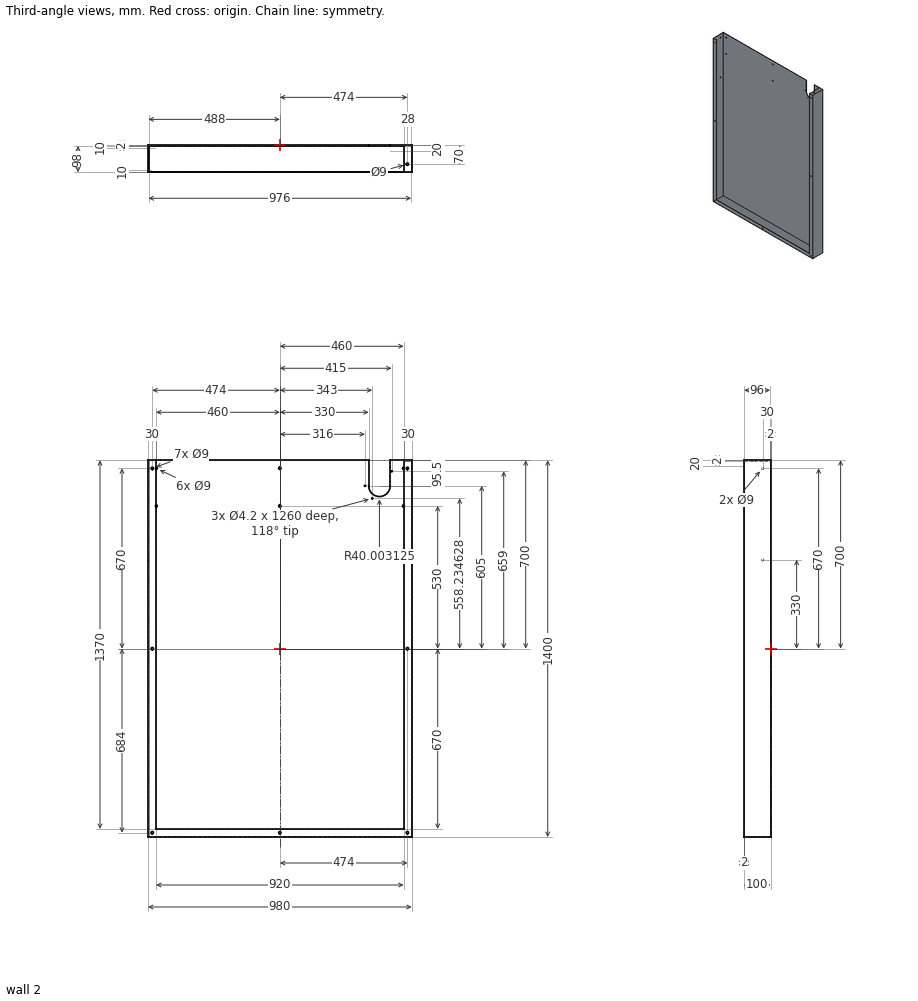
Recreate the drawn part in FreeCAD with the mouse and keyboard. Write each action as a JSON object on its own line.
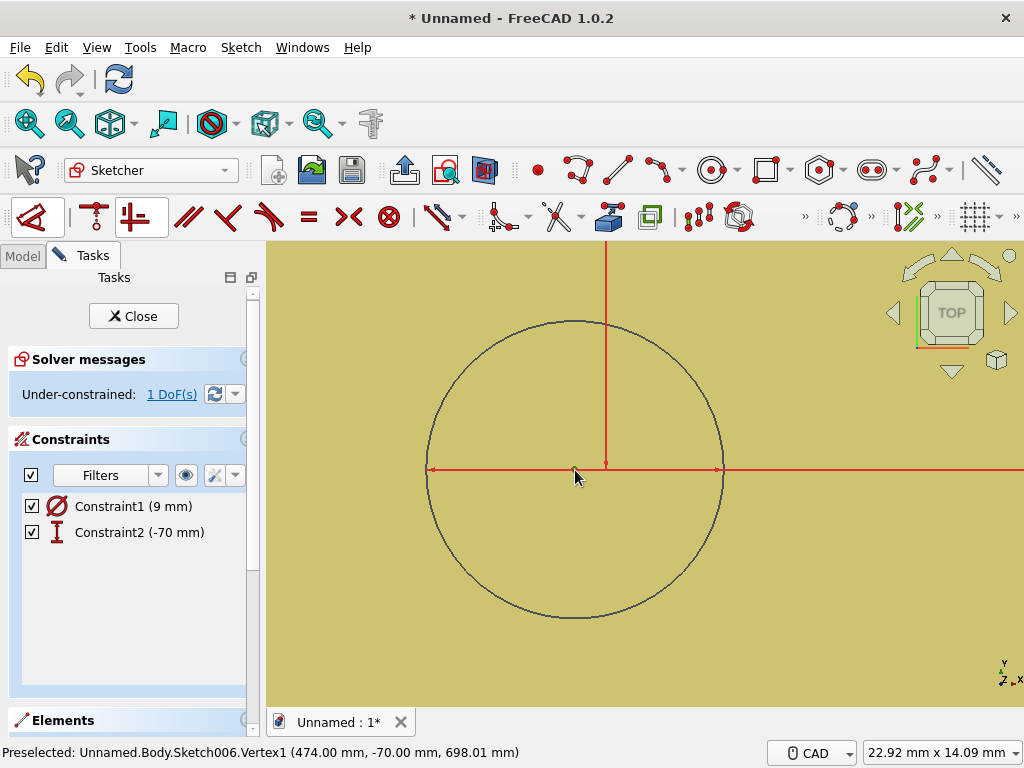
{"action": "left_click", "coordinate": [58, 218]}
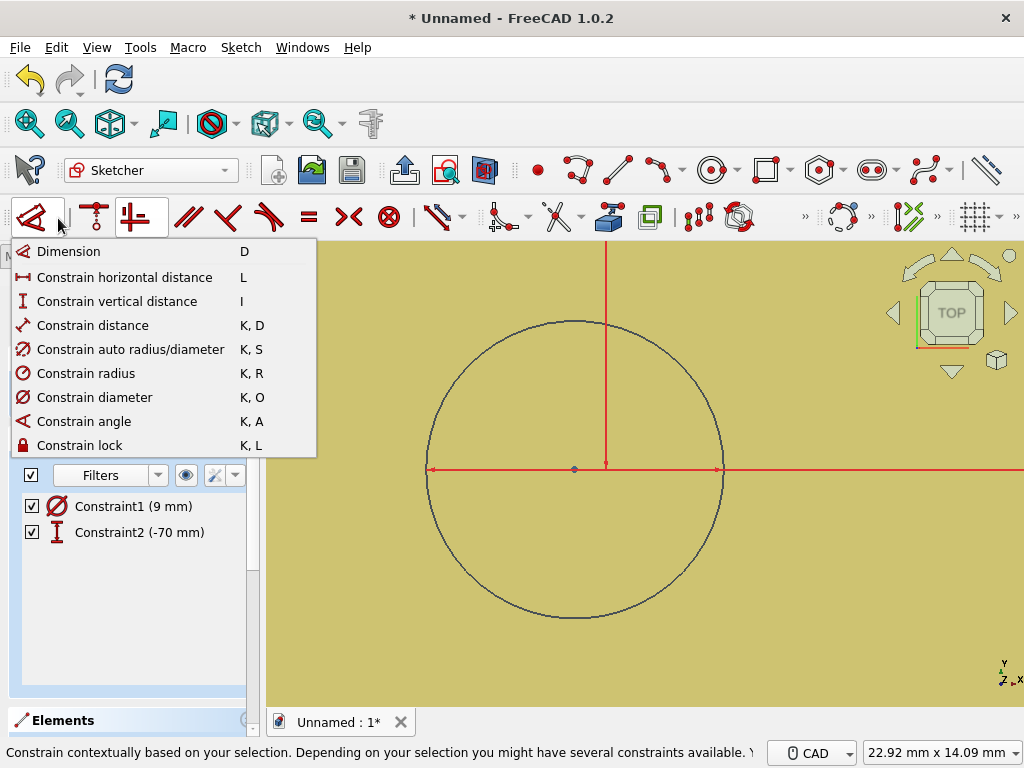
{"action": "left_click", "coordinate": [164, 277]}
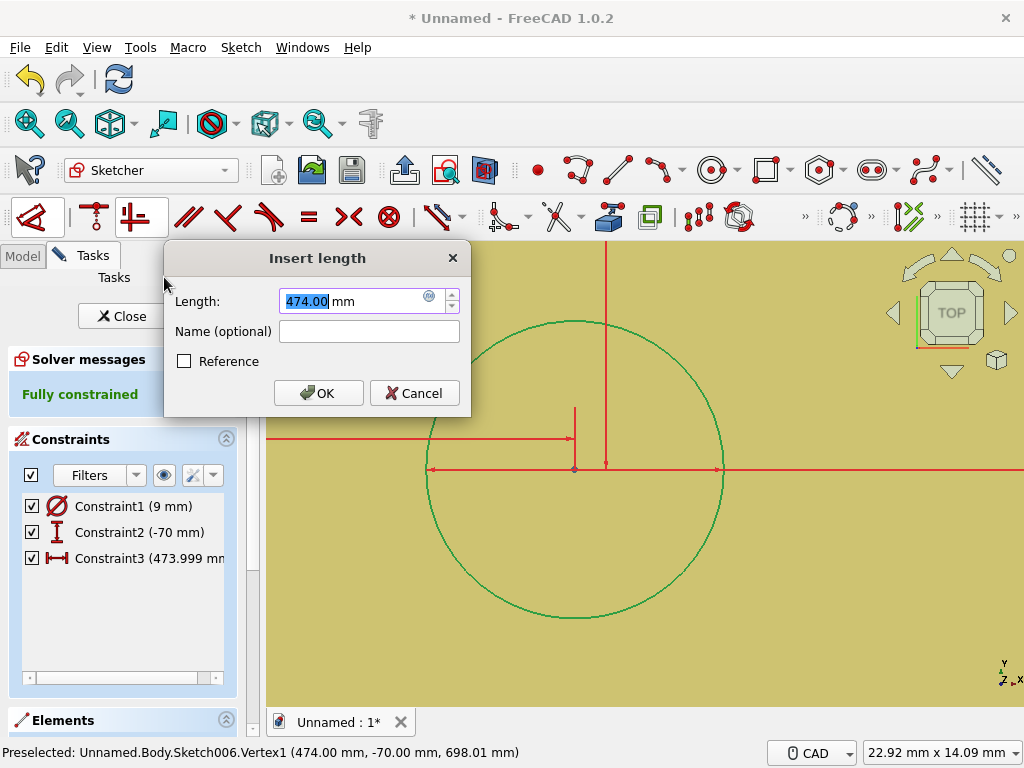
{"action": "type", "text": "474"}
{"action": "key", "text": "Return"}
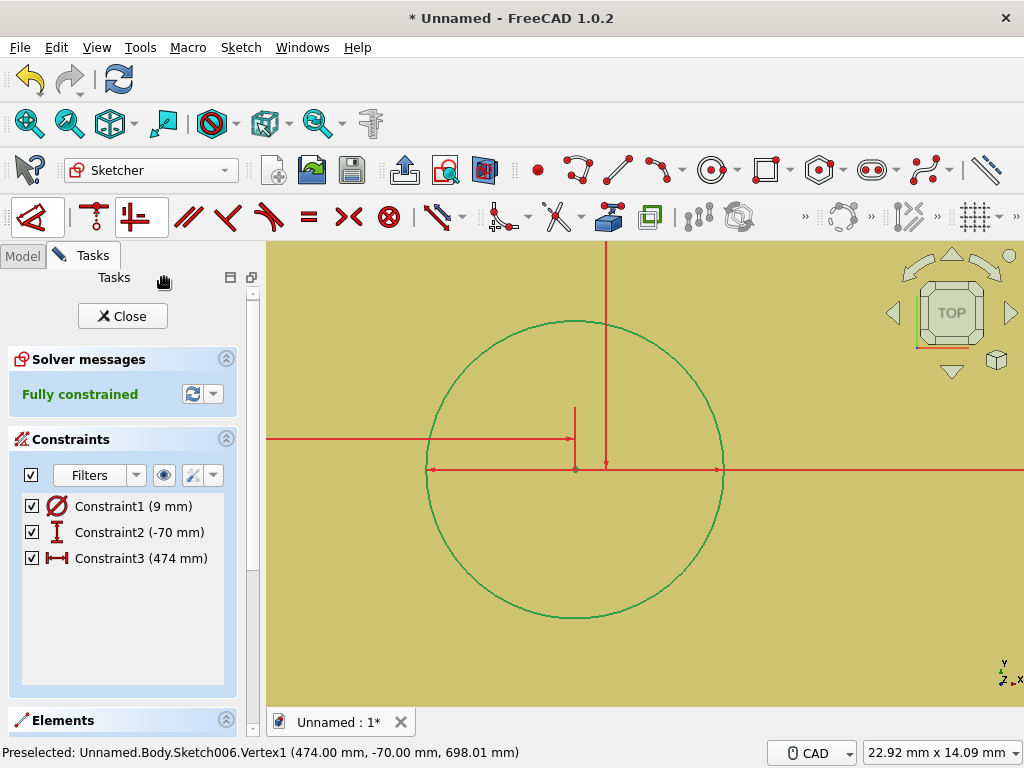
{"action": "left_click", "coordinate": [123, 316]}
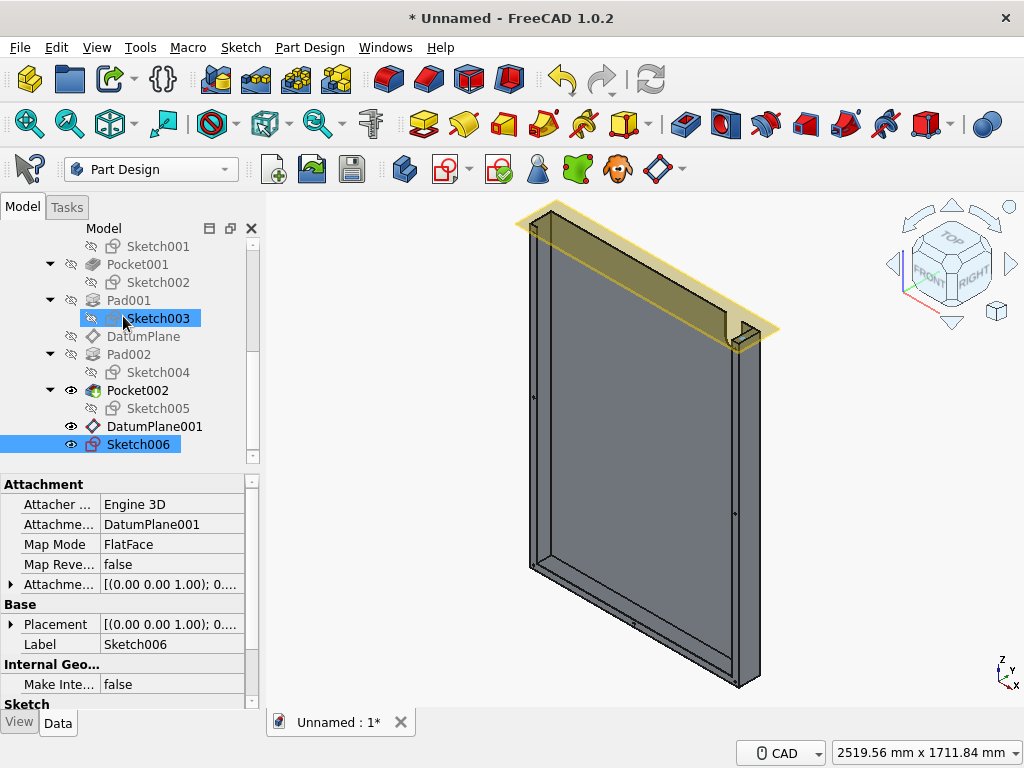
{"action": "left_click", "coordinate": [686, 124]}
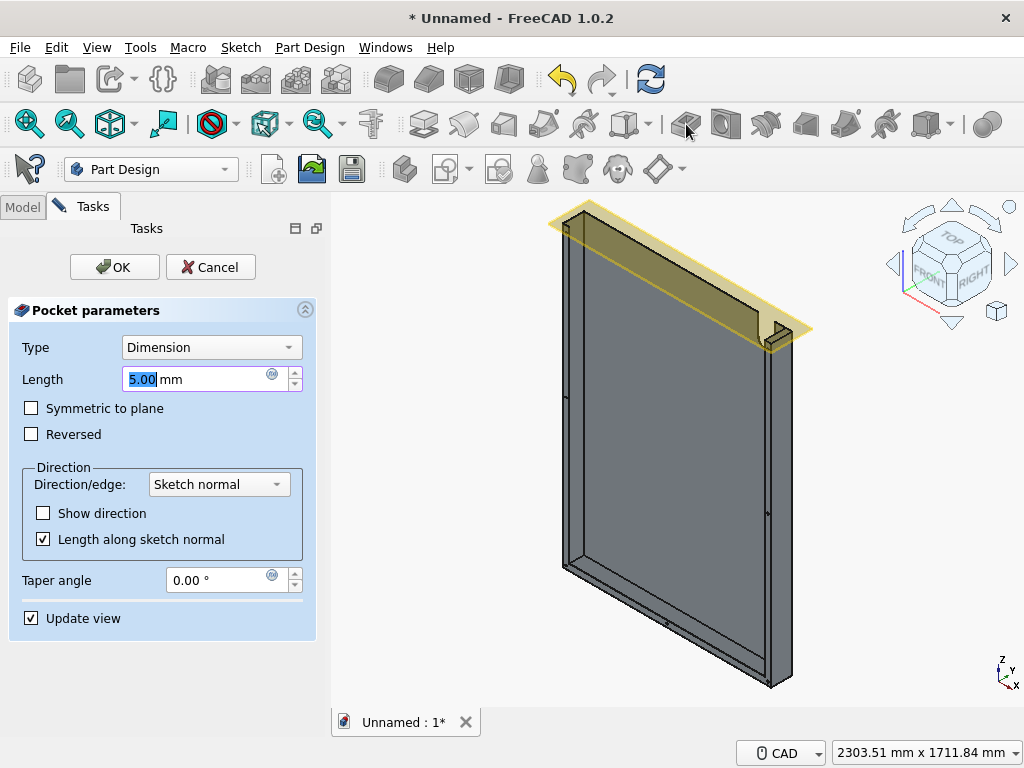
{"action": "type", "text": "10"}
{"action": "key", "text": "Tab"}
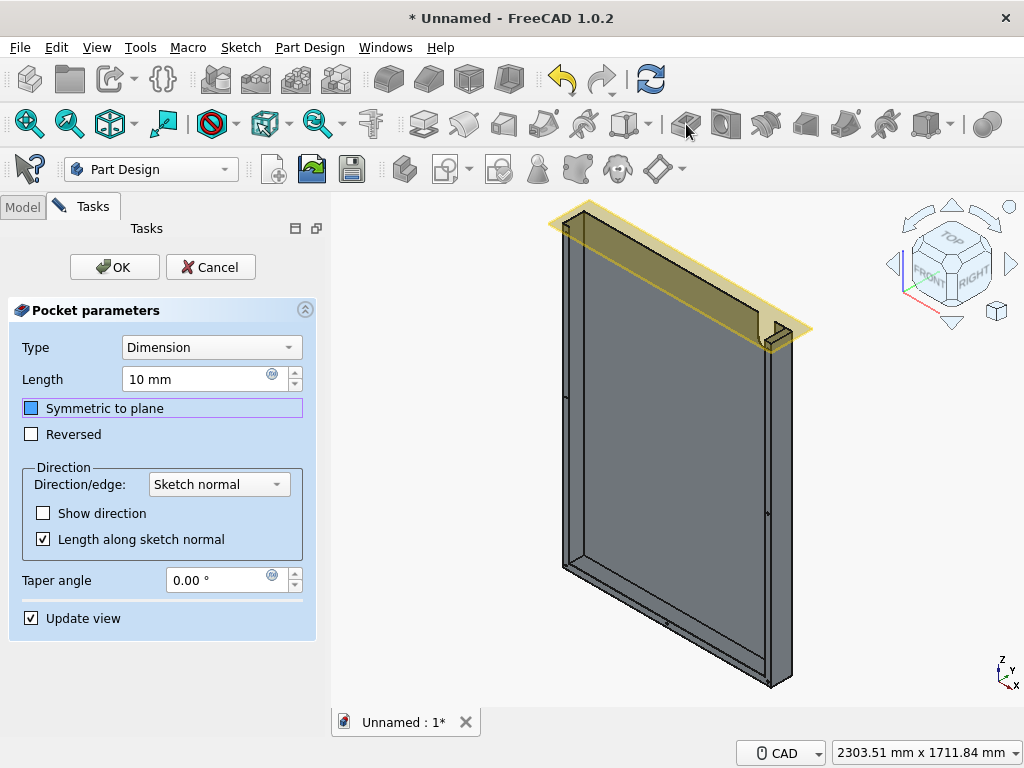
{"action": "left_click", "coordinate": [30, 434]}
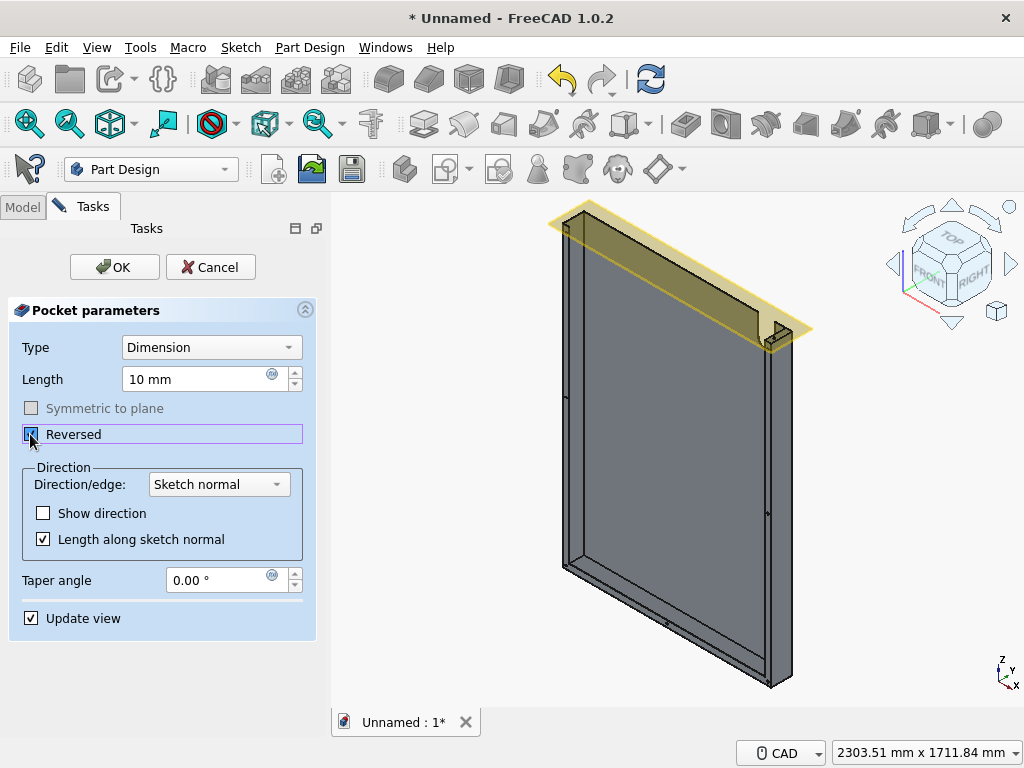
{"action": "left_click", "coordinate": [115, 267]}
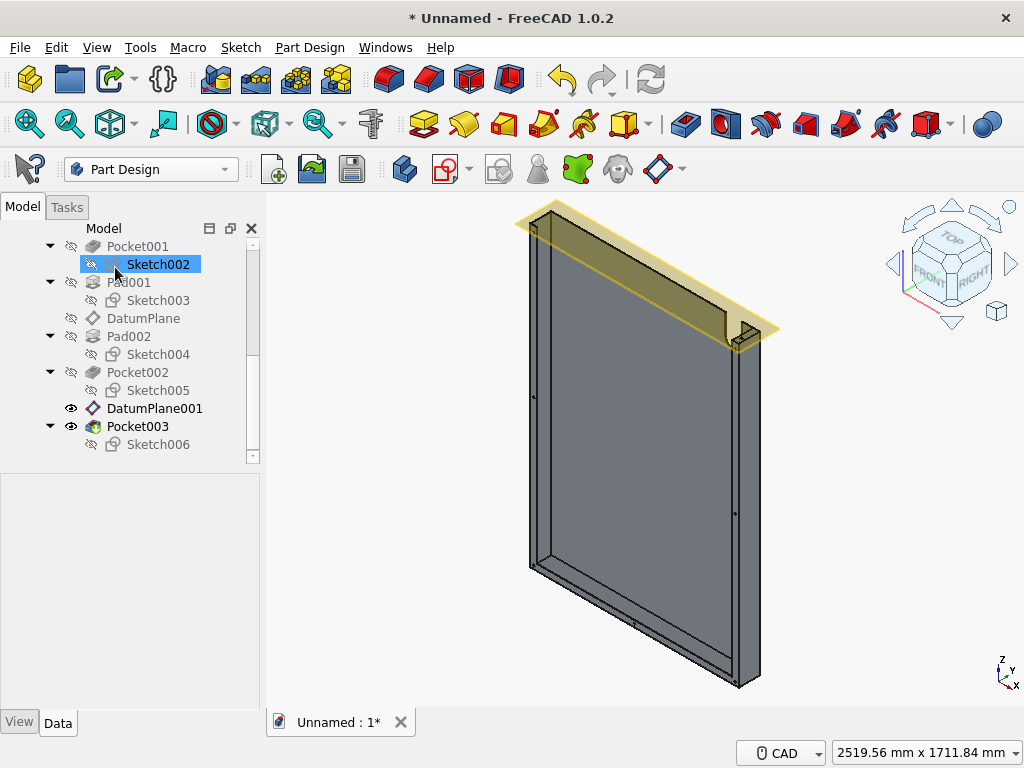
{"action": "left_click", "coordinate": [116, 408]}
{"action": "key", "text": "space"}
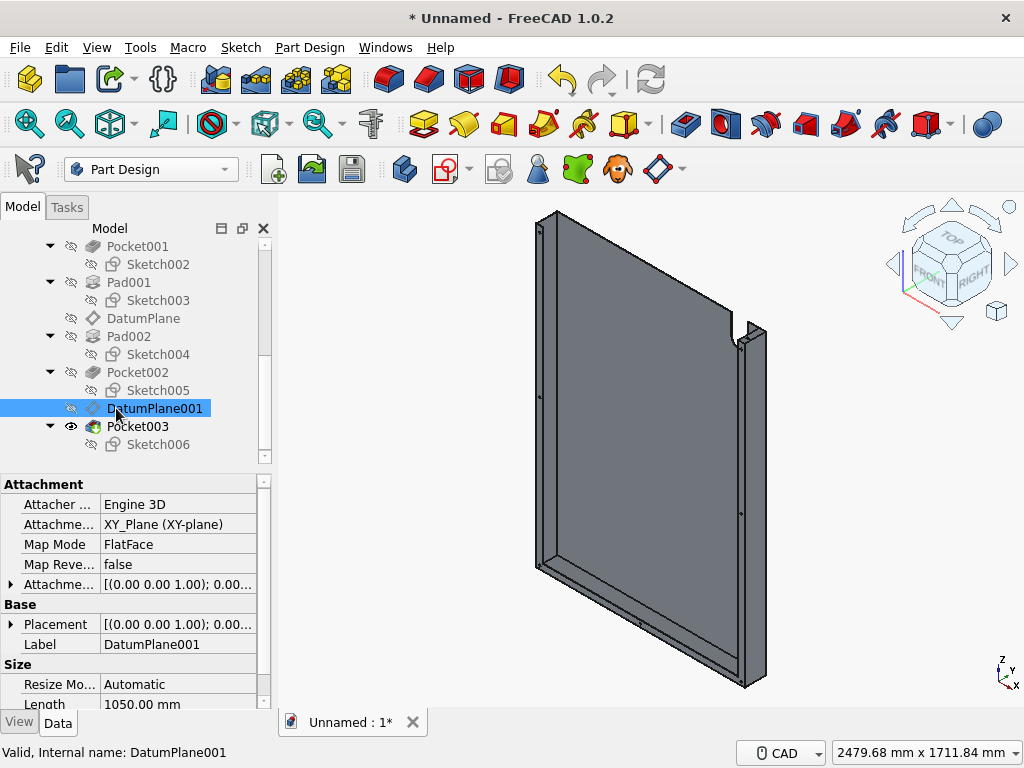
{"action": "scroll", "coordinate": [140, 350], "scroll_direction": "down", "scroll_amount": 3}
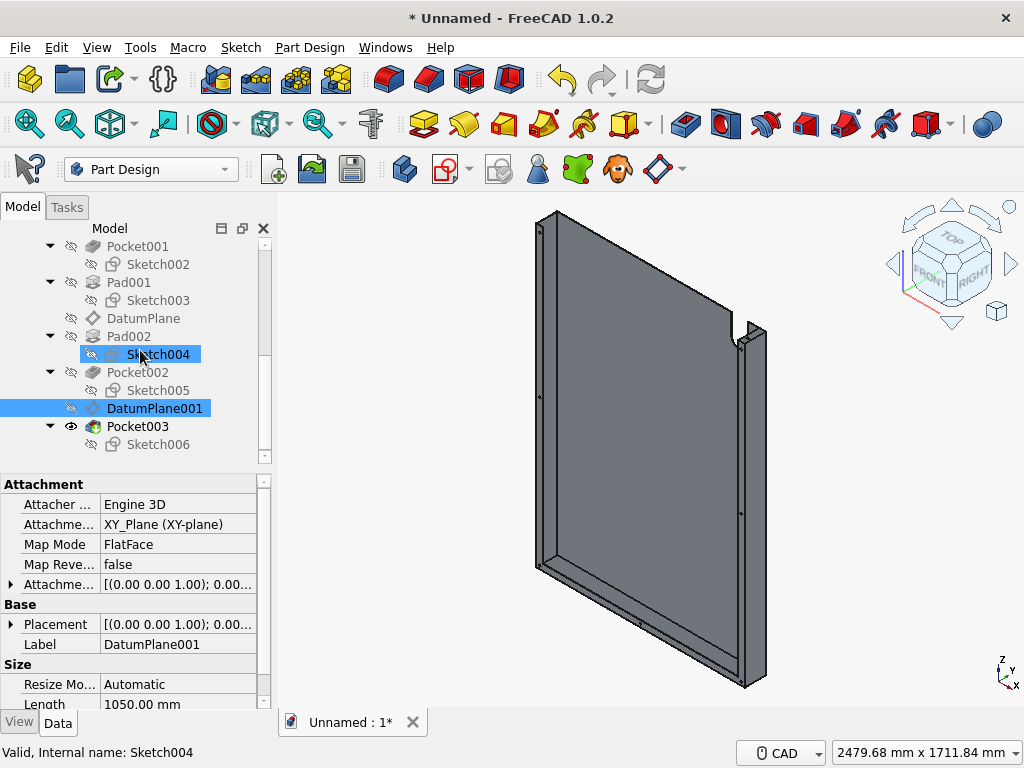
{"action": "scroll", "coordinate": [140, 350], "scroll_direction": "up", "scroll_amount": 15}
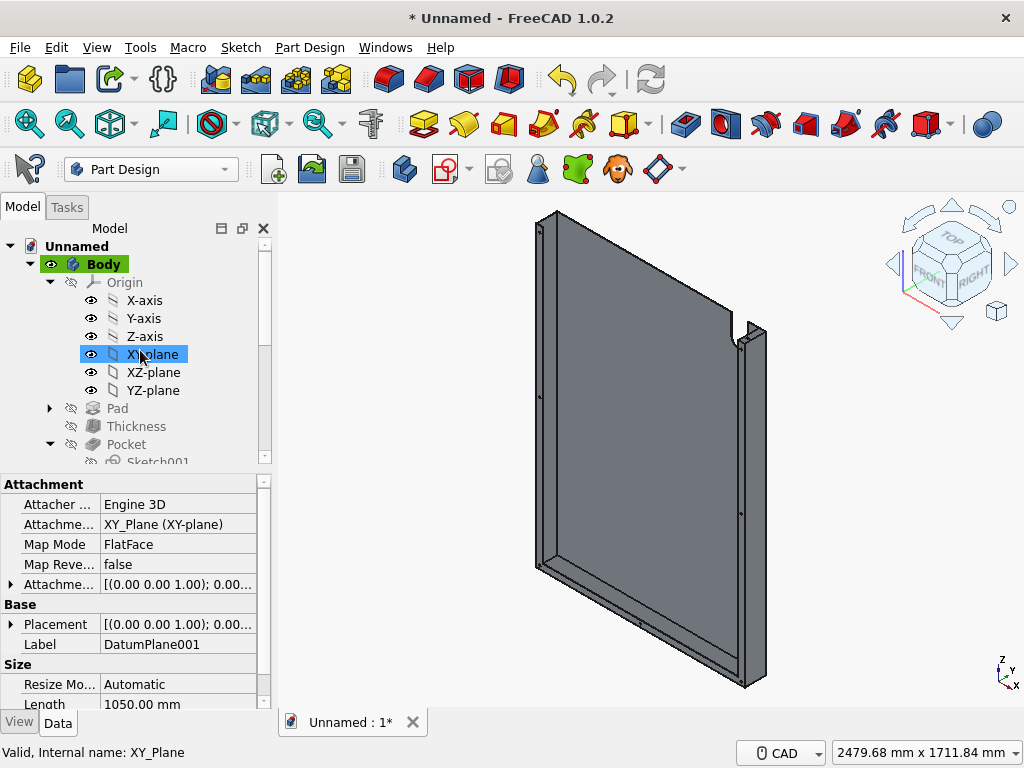
{"action": "left_click", "coordinate": [136, 390]}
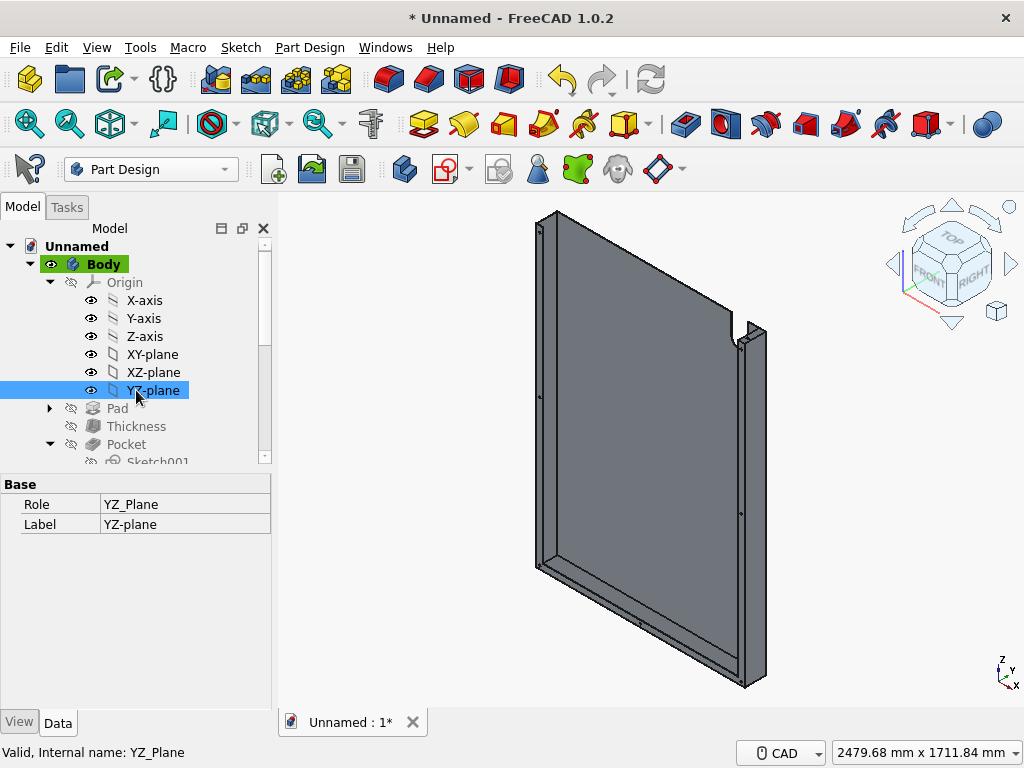
{"action": "left_click", "coordinate": [658, 170]}